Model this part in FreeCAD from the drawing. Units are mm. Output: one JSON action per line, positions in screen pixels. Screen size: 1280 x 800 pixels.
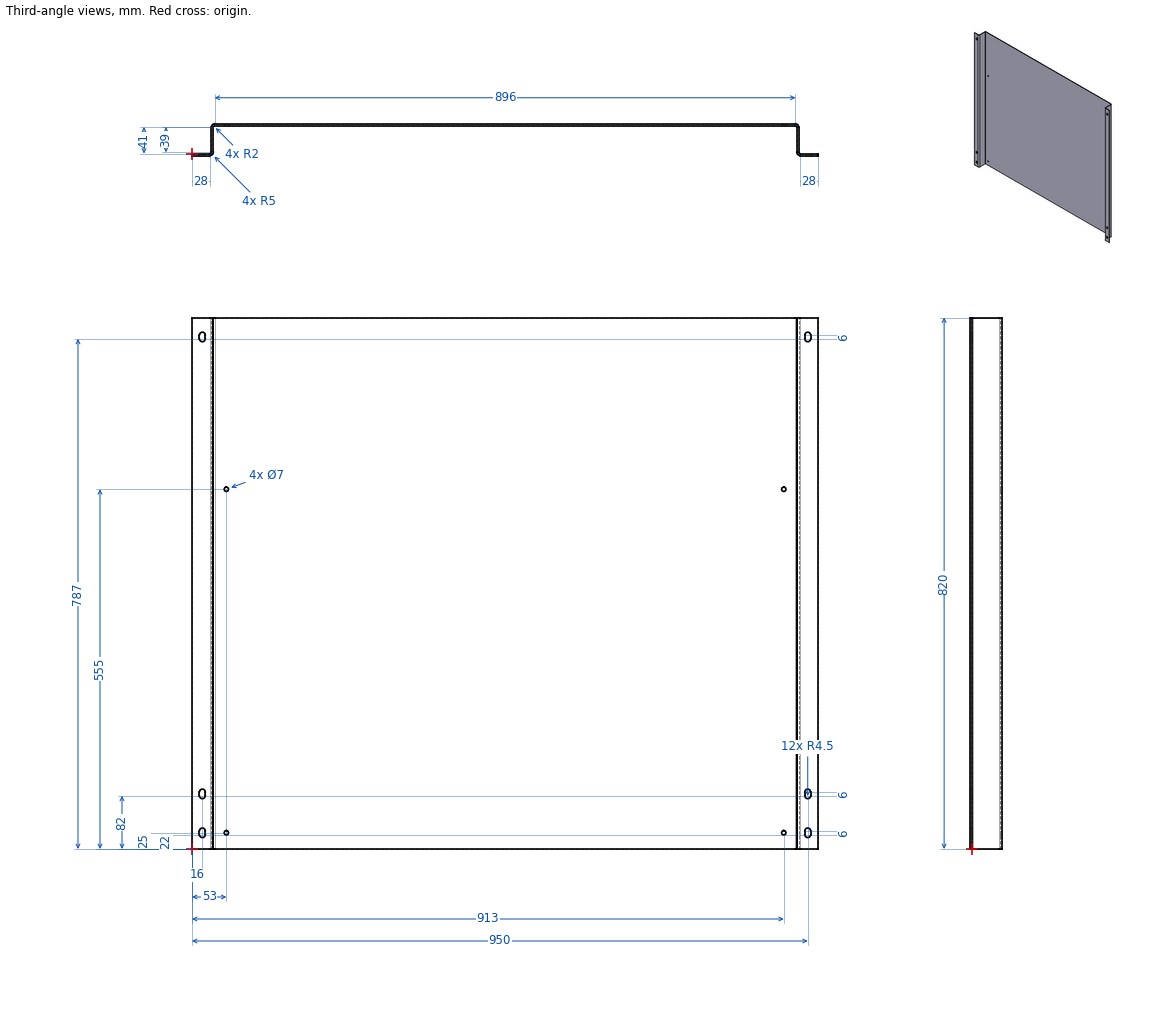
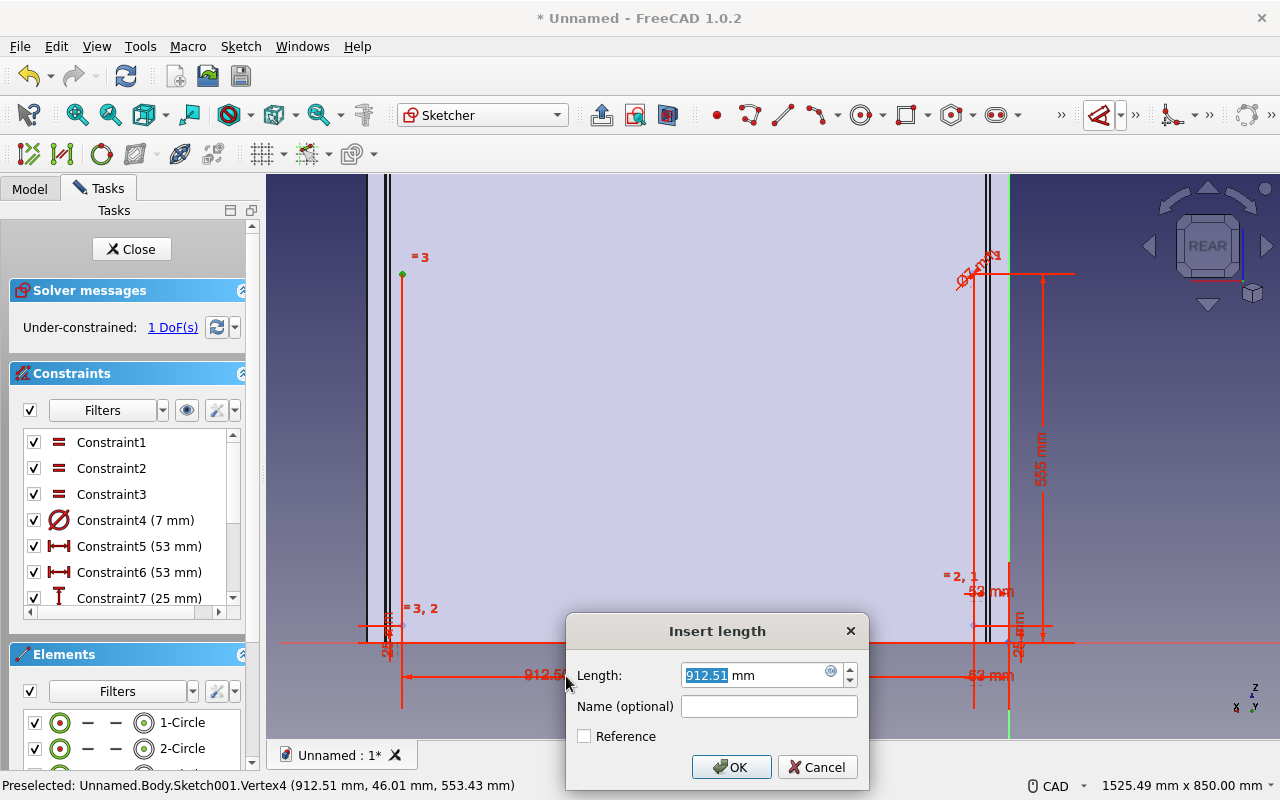
{"action": "type", "text": "913"}
{"action": "key", "text": "Return"}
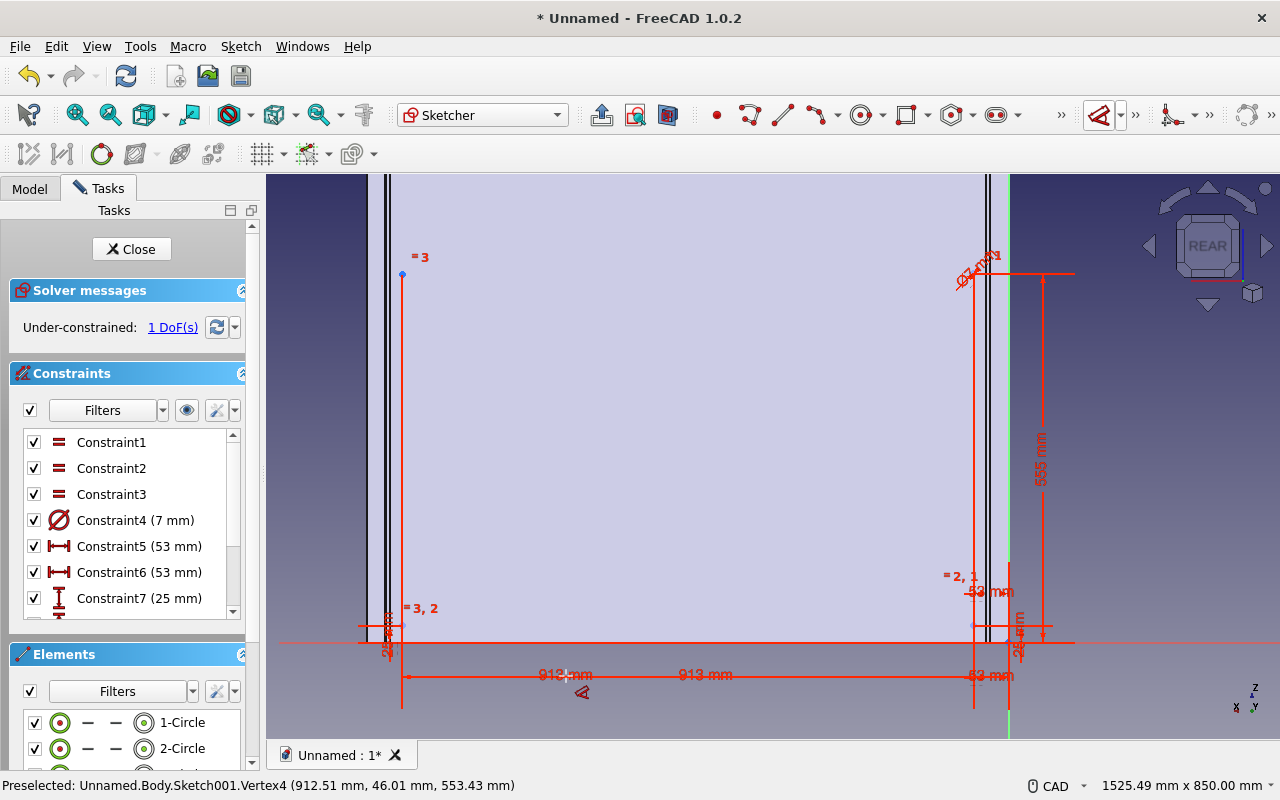
{"action": "left_click", "coordinate": [402, 275]}
{"action": "left_click", "coordinate": [1043, 374]}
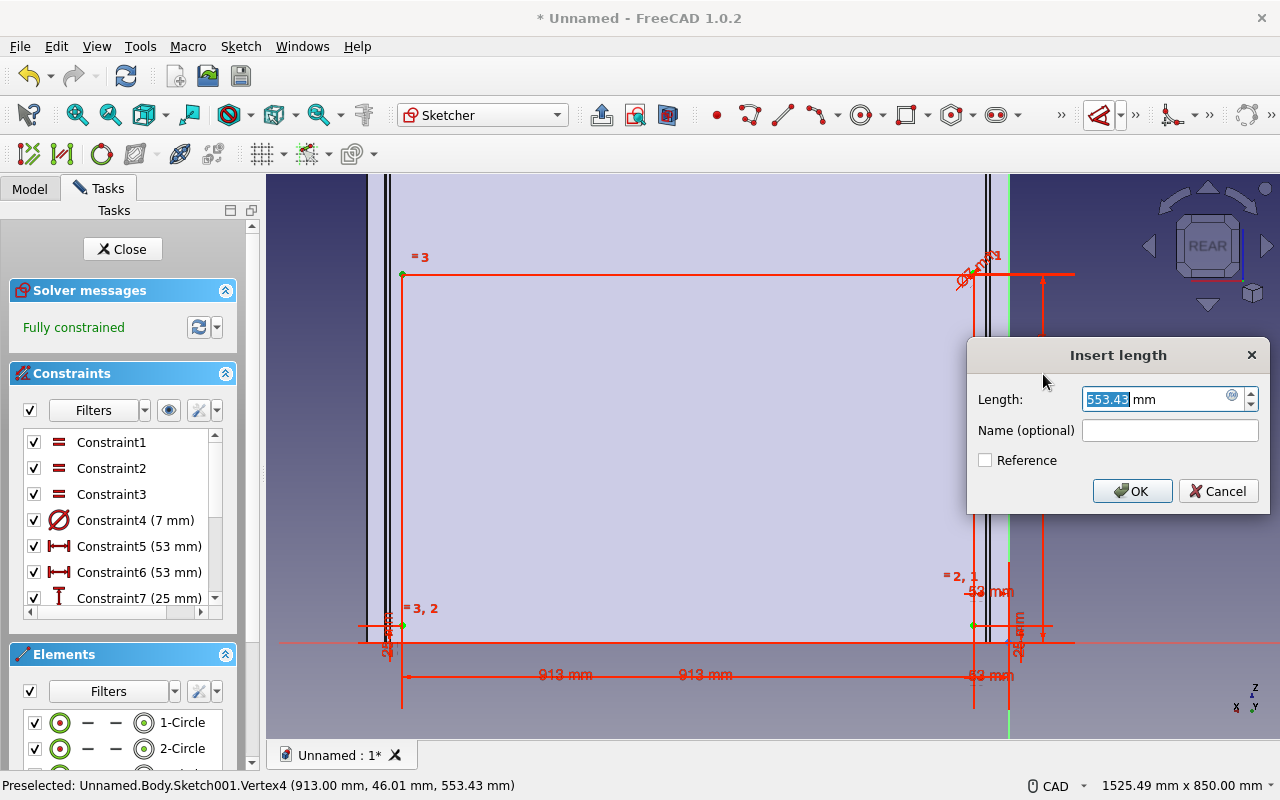
{"action": "type", "text": "555"}
{"action": "key", "text": "Return"}
{"action": "key", "text": "Escape"}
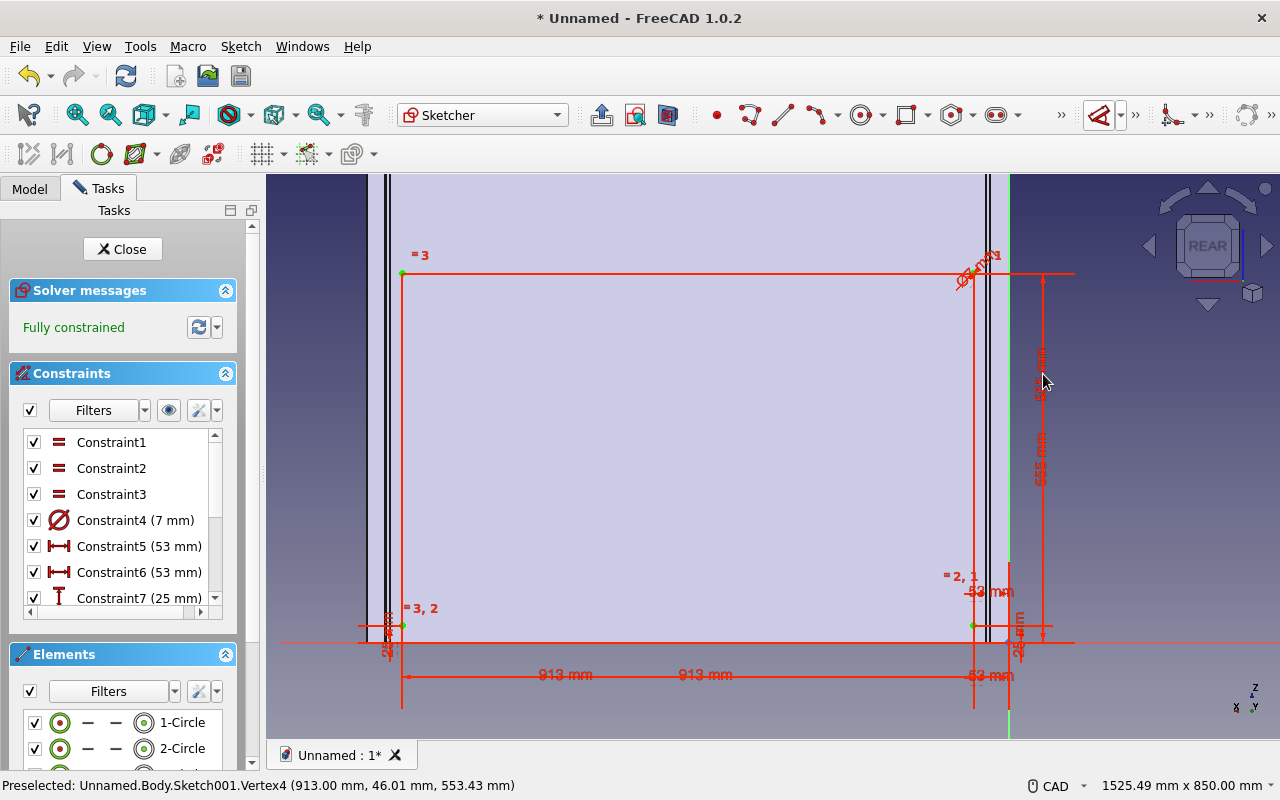
{"action": "left_click", "coordinate": [123, 249]}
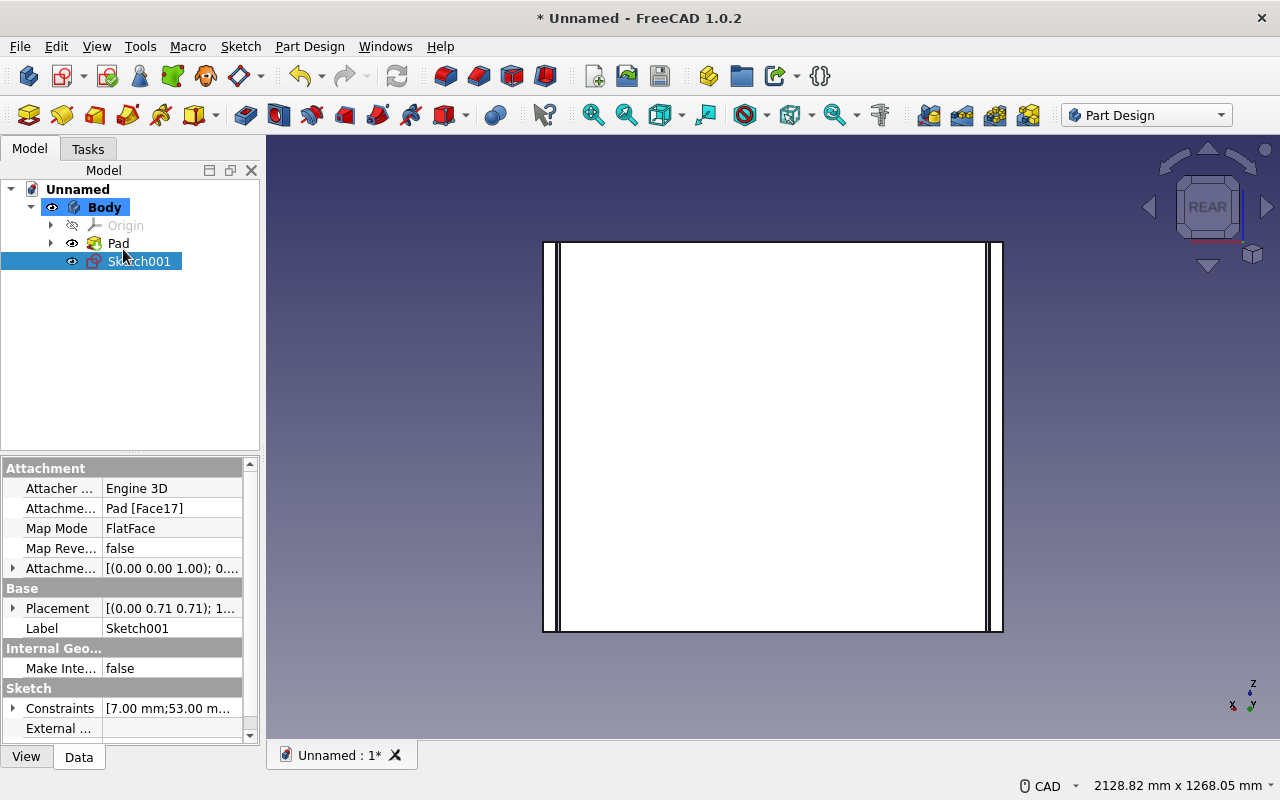
{"action": "left_click", "coordinate": [246, 116]}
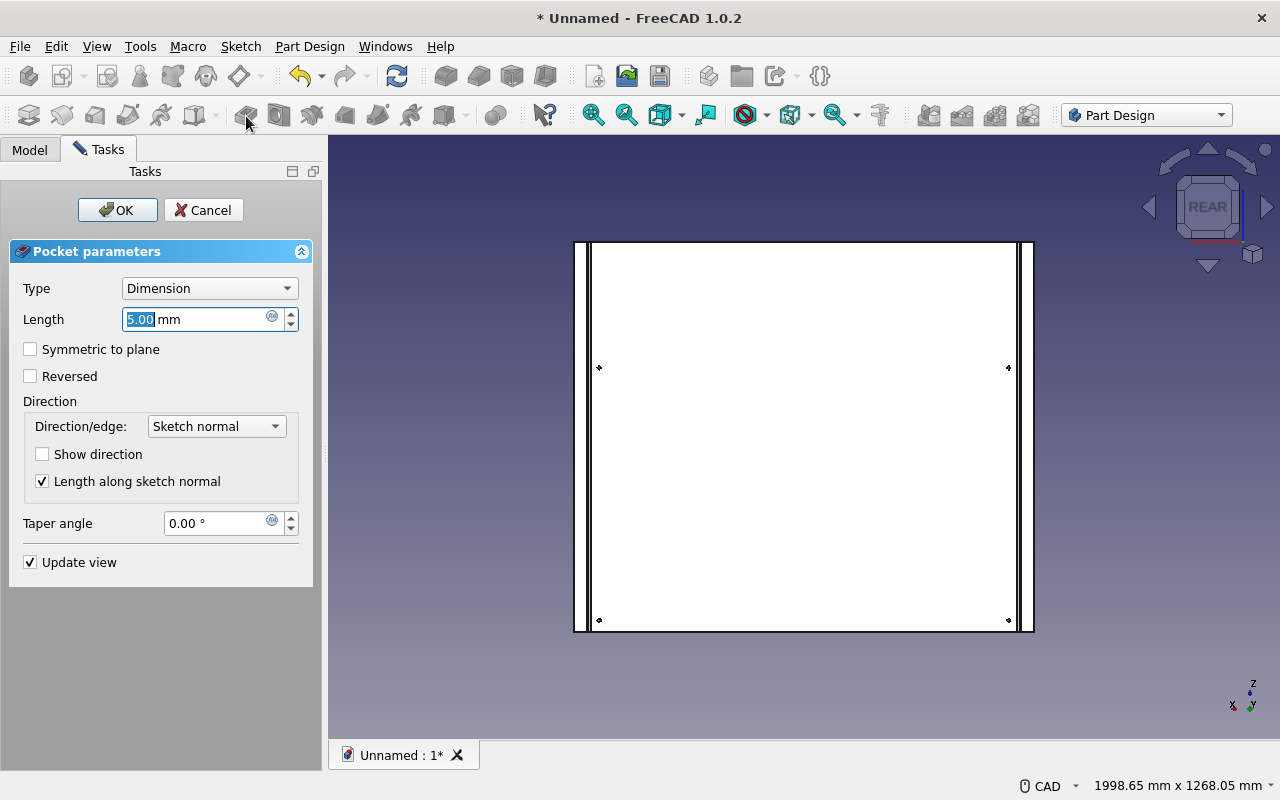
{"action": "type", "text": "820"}
{"action": "key", "text": "Tab"}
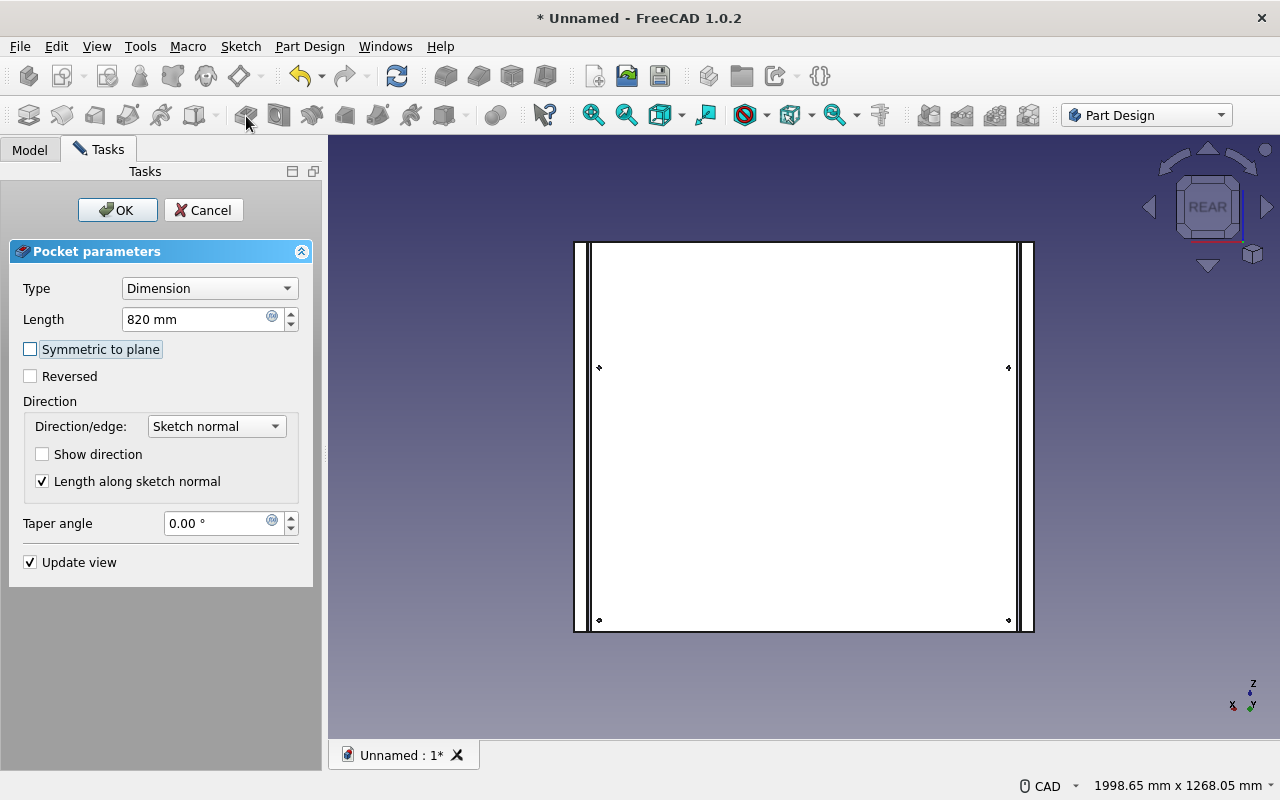
{"action": "left_click", "coordinate": [118, 210]}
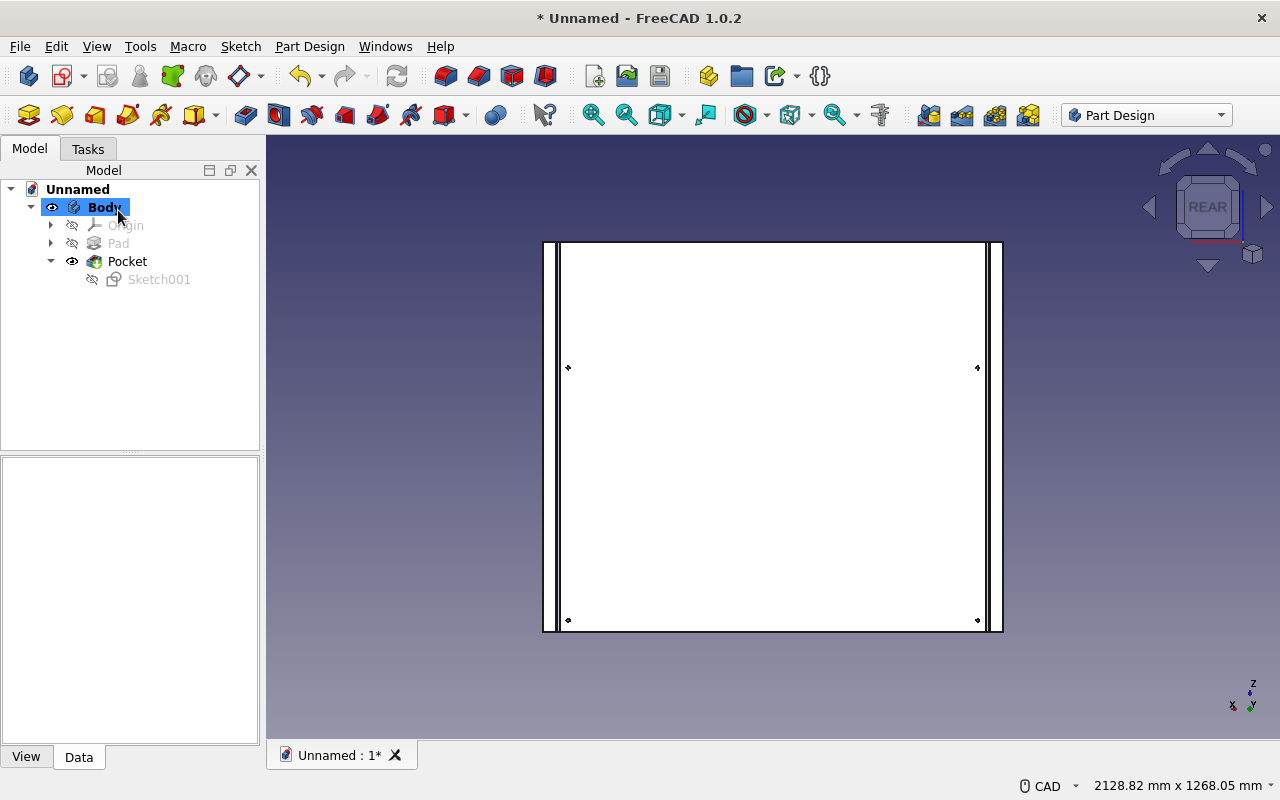
{"action": "left_click", "coordinate": [62, 76]}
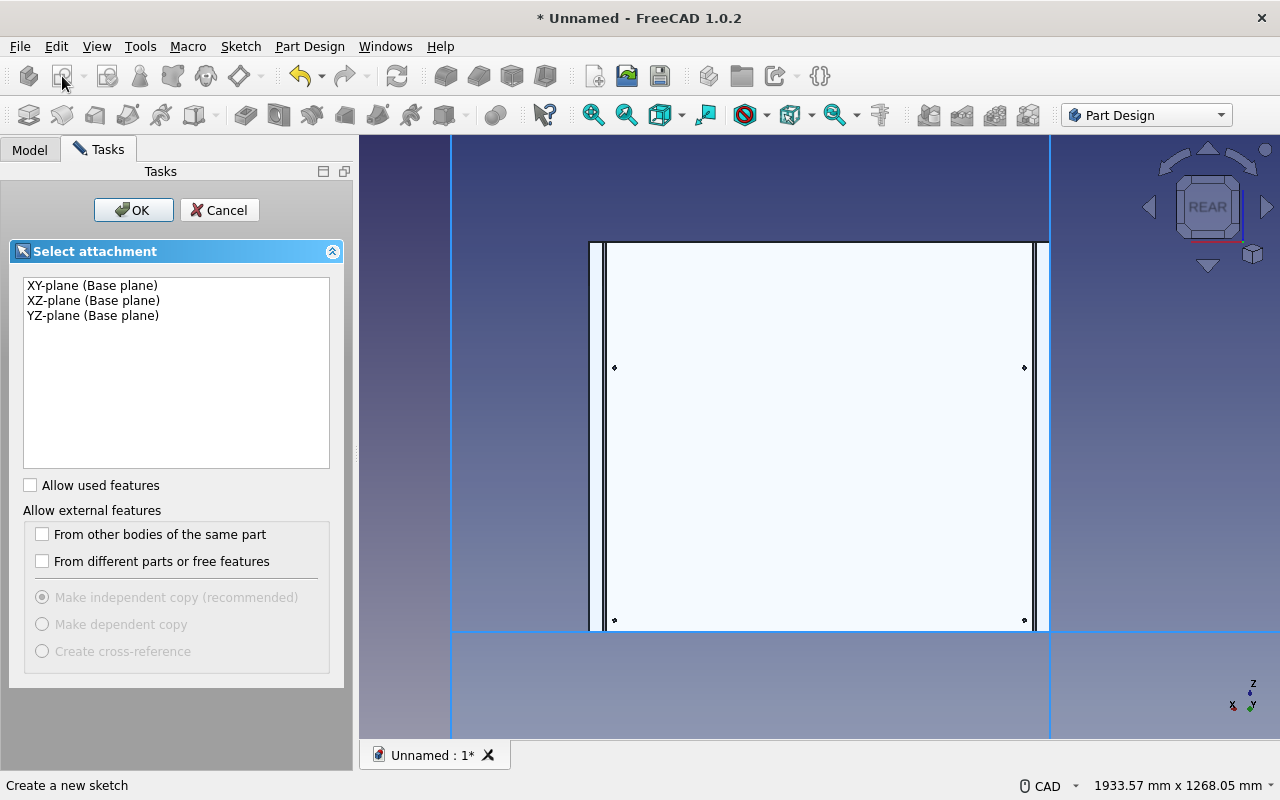
{"action": "left_click", "coordinate": [84, 300]}